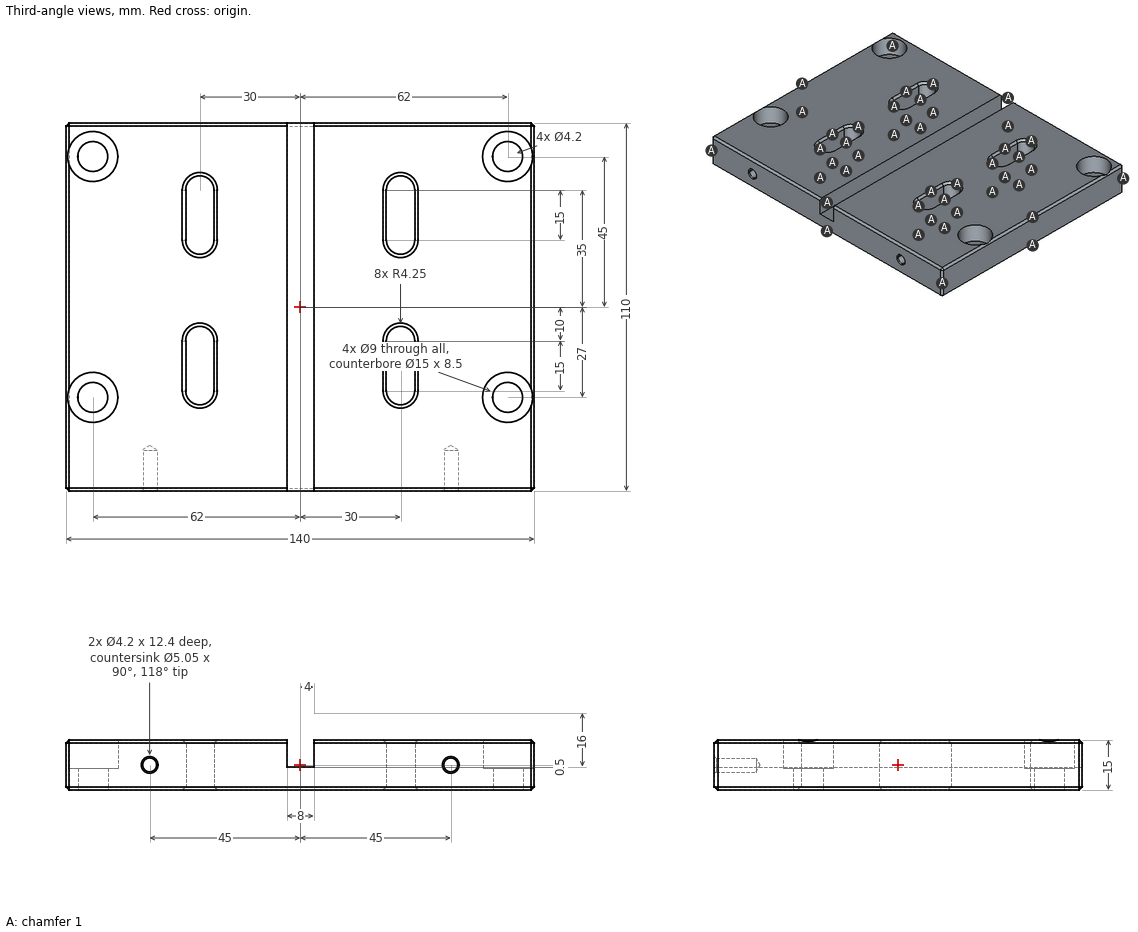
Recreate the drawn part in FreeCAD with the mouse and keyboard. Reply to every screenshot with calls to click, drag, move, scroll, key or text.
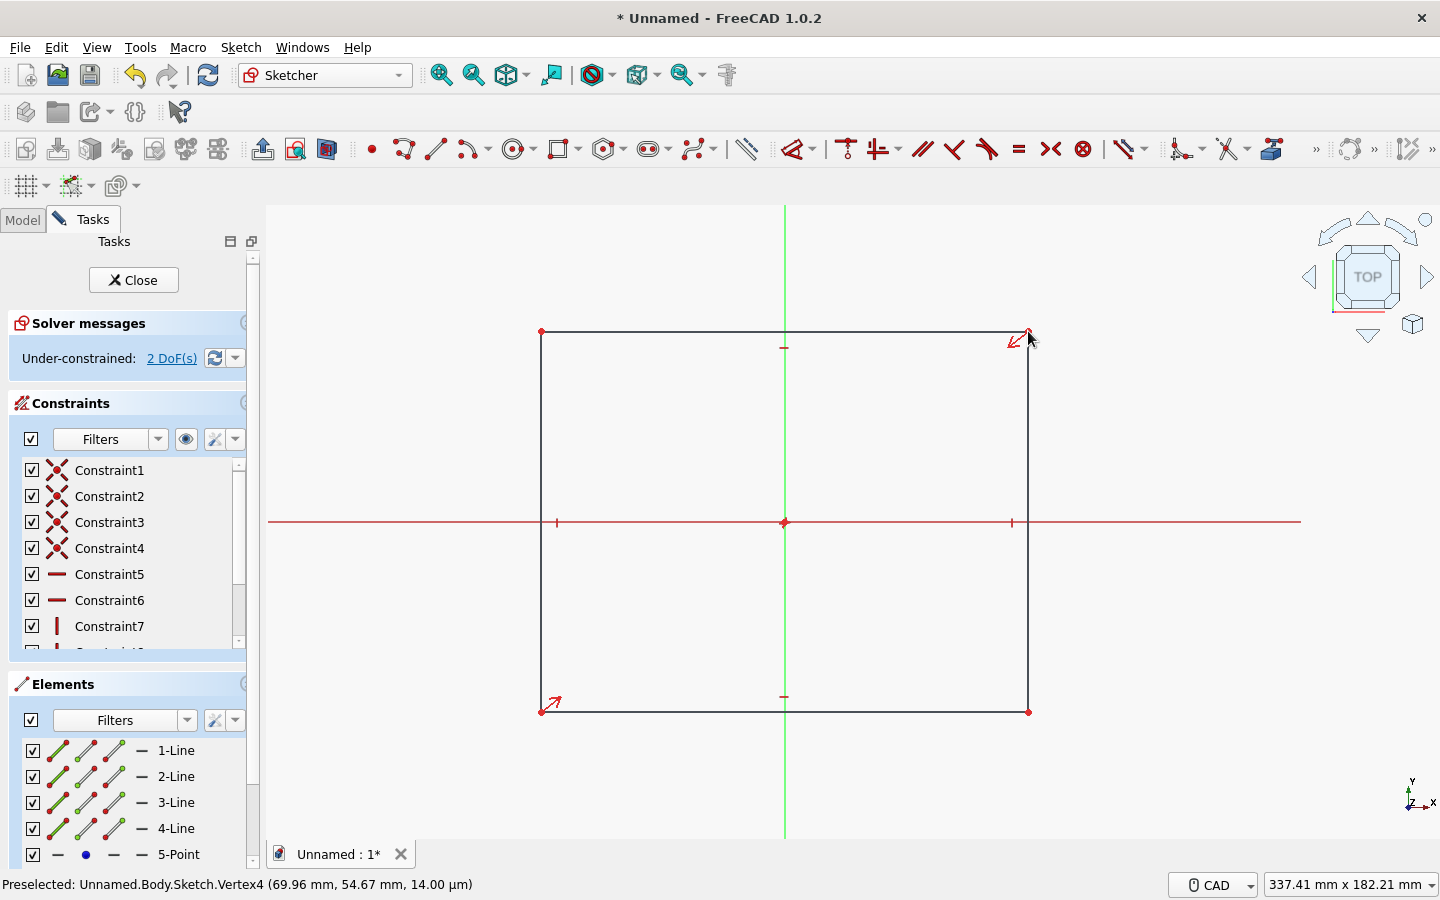
click(792, 150)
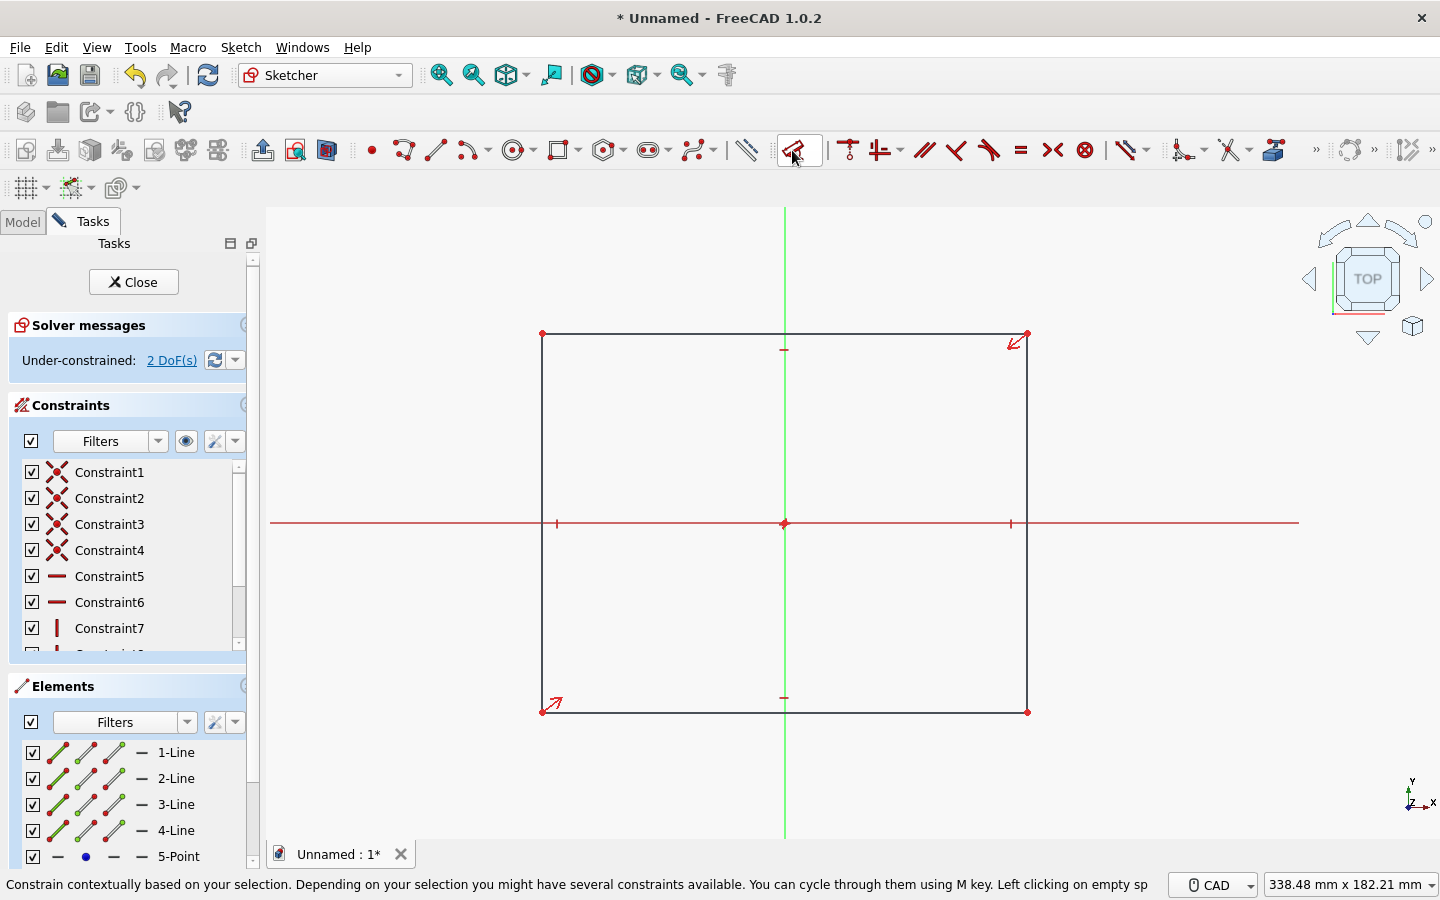
click(688, 713)
click(673, 747)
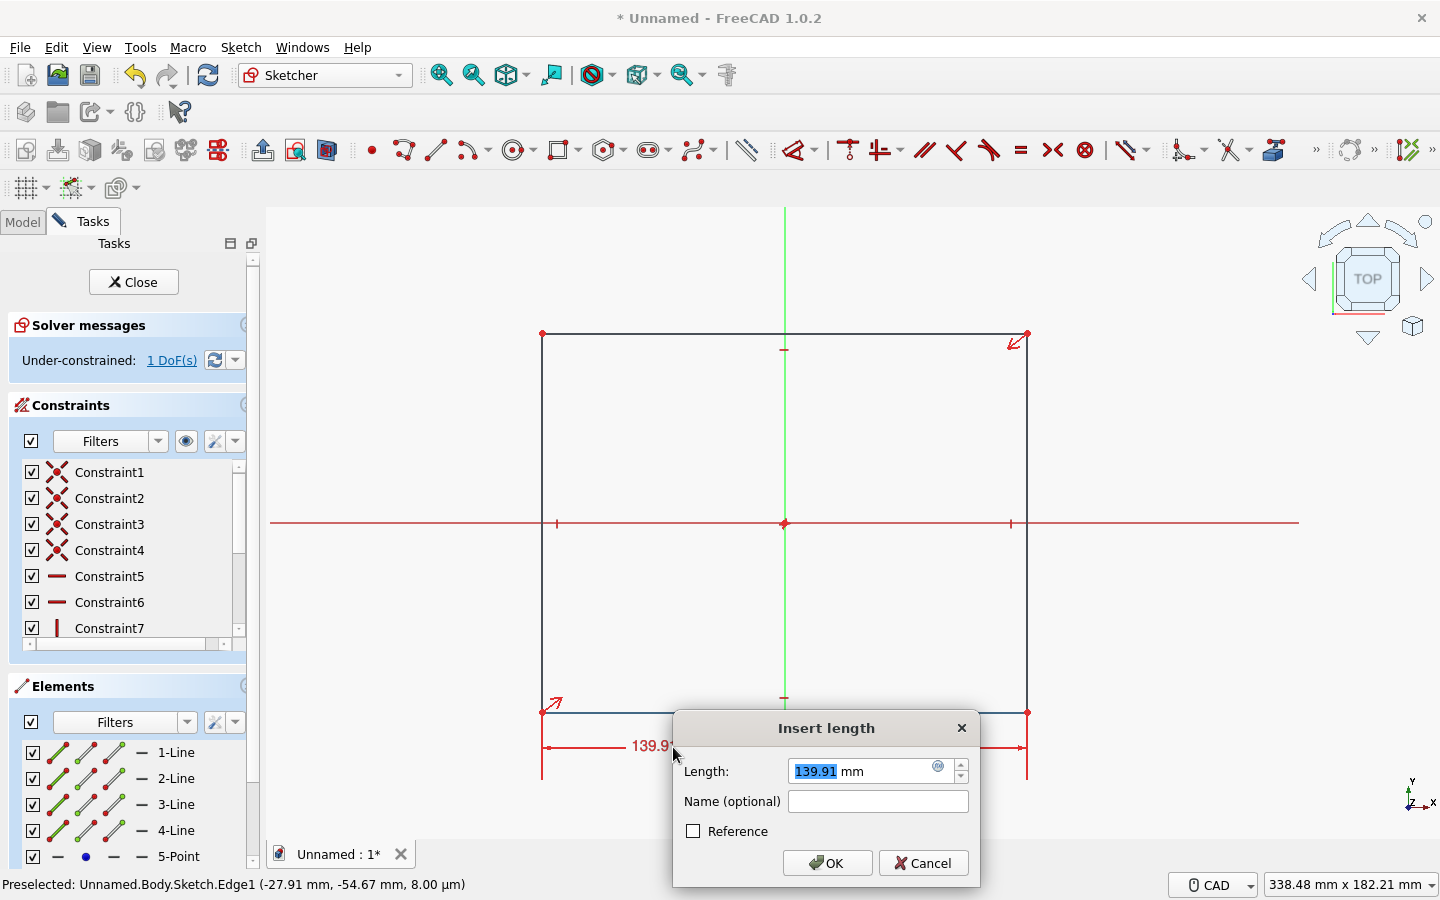
text(140)
key(Return)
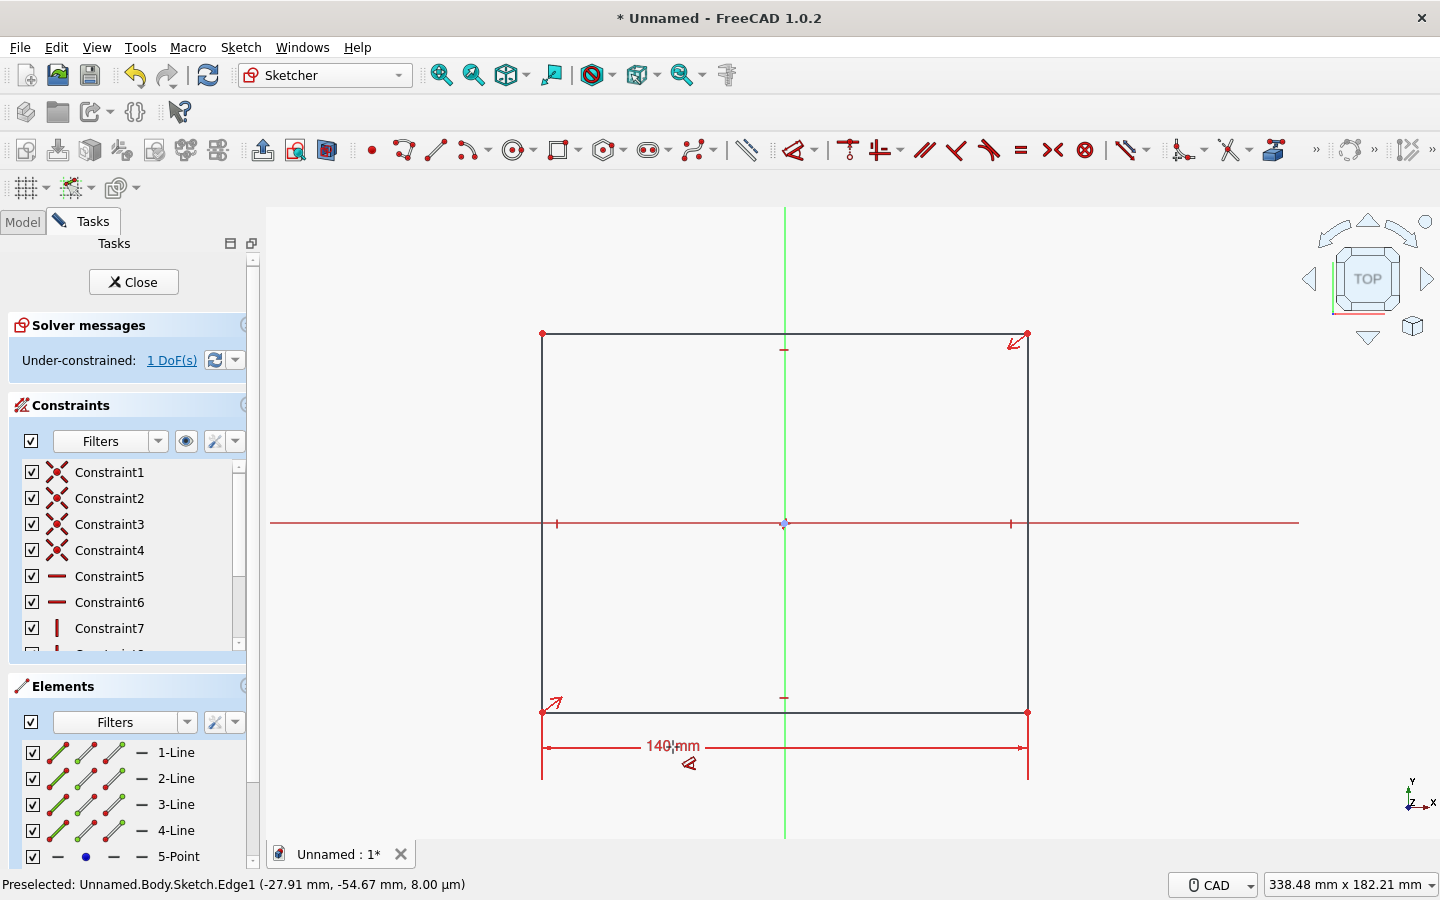
click(1028, 599)
click(1062, 436)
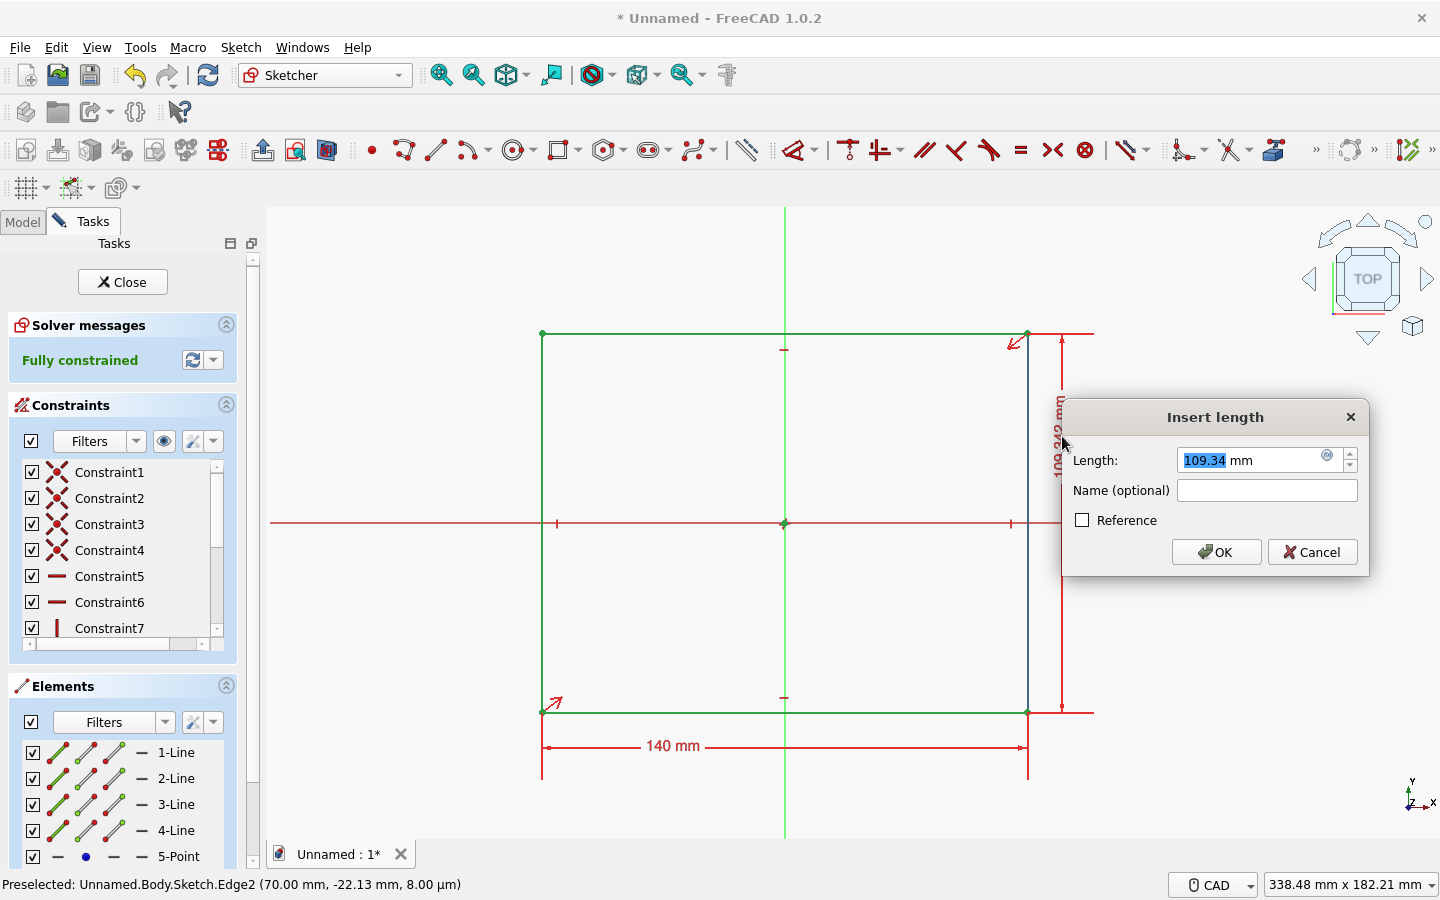
text(110)
key(Return)
key(Escape)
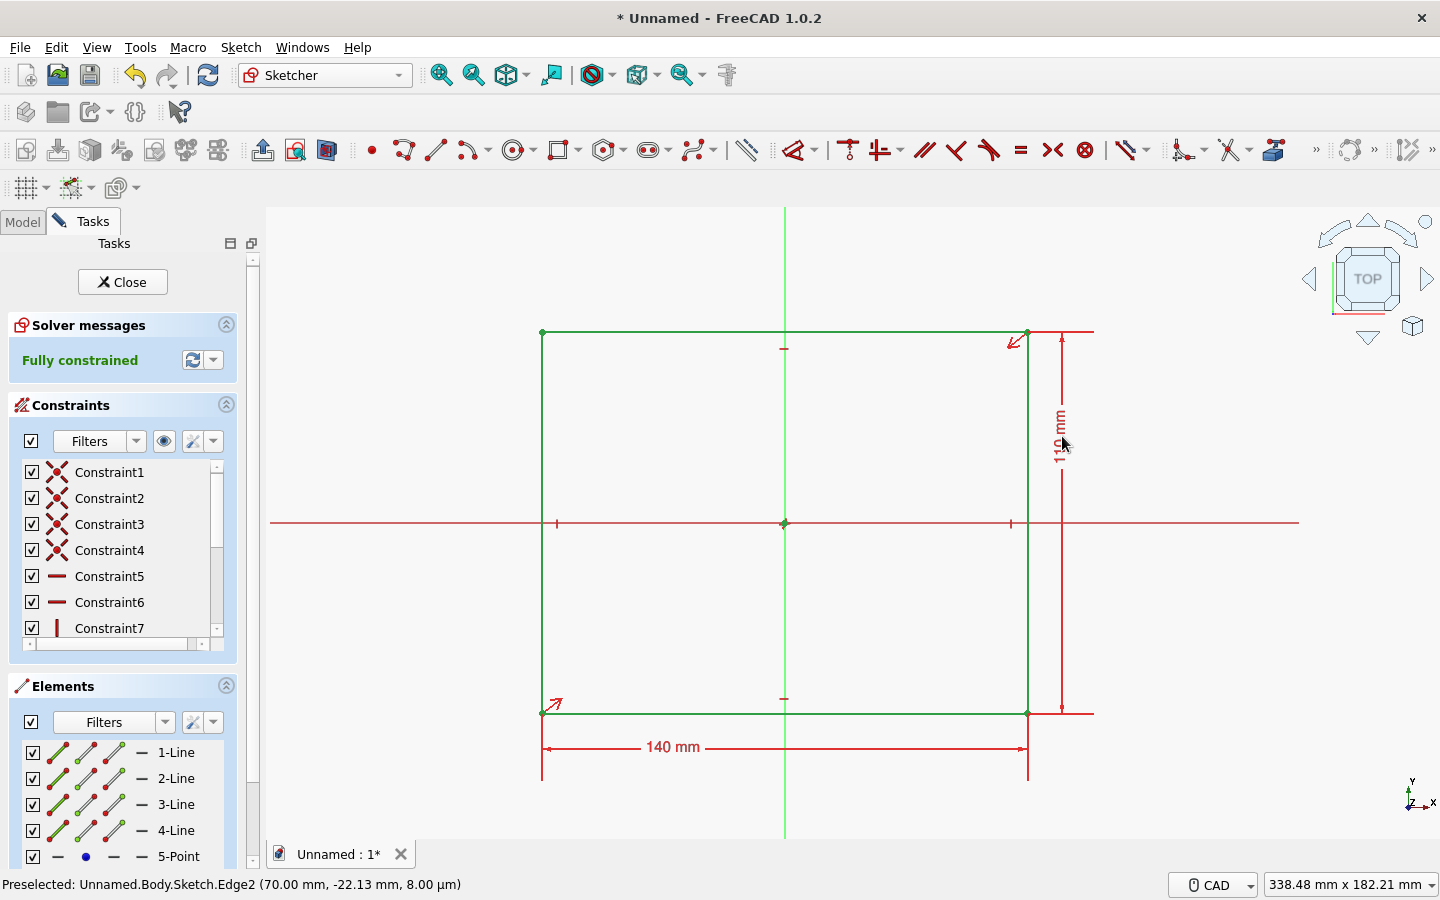
click(123, 282)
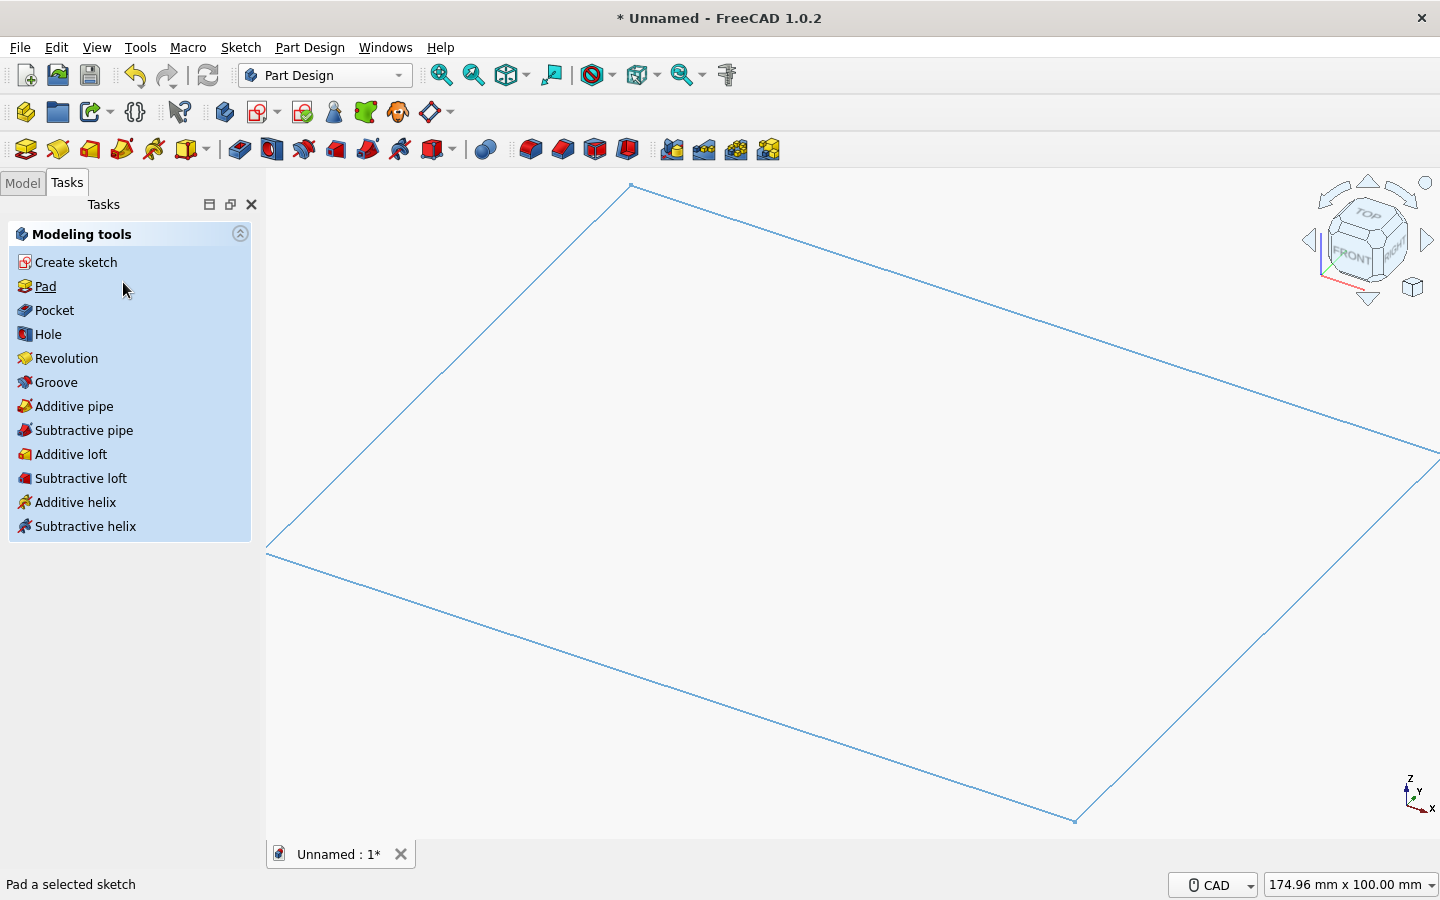
click(26, 150)